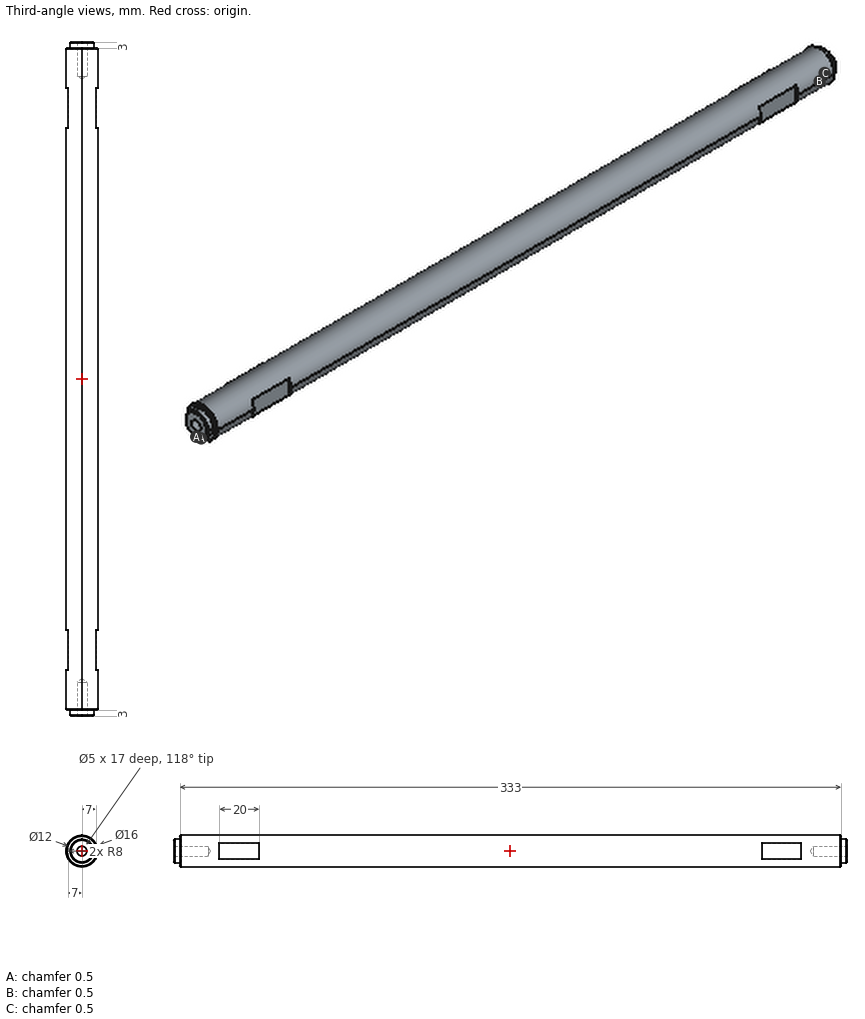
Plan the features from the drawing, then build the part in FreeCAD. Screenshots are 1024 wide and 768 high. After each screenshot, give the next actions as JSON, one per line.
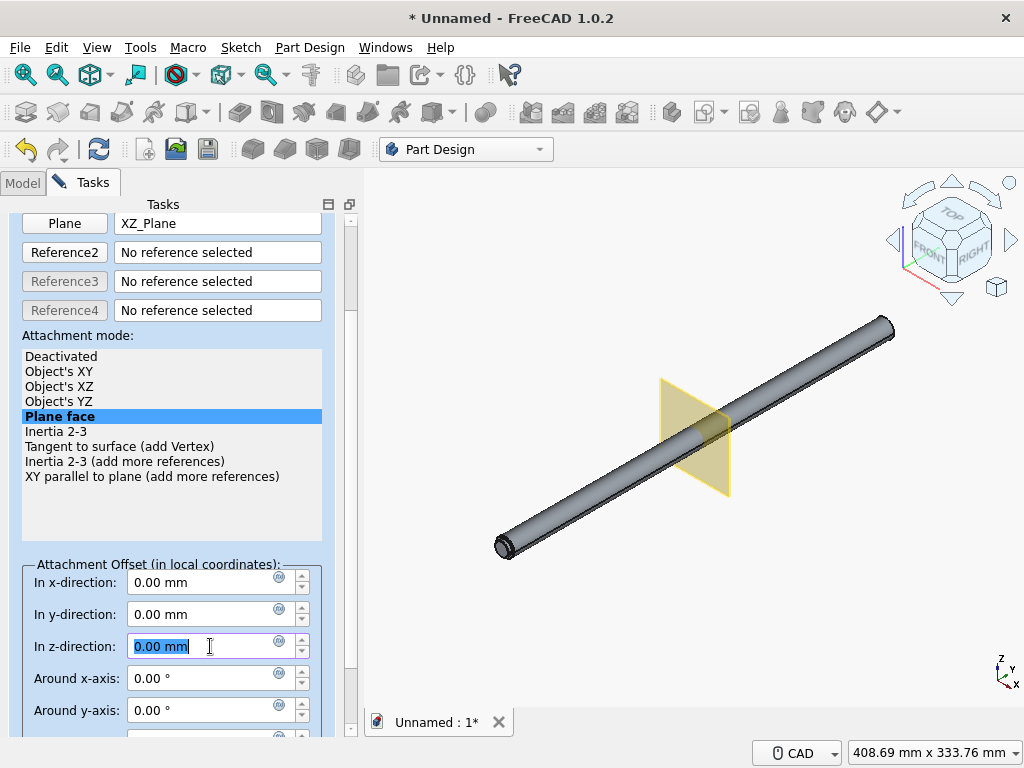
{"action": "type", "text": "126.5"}
{"action": "key", "text": "Tab"}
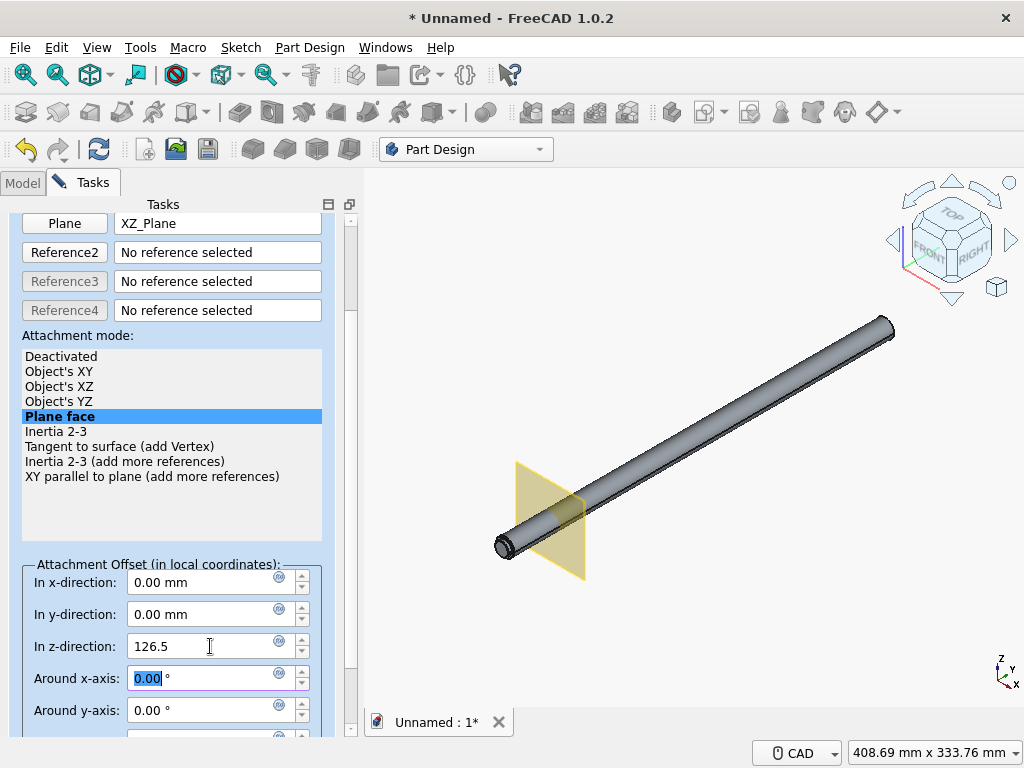
{"action": "scroll", "coordinate": [351, 475], "scroll_direction": "up", "scroll_amount": 3}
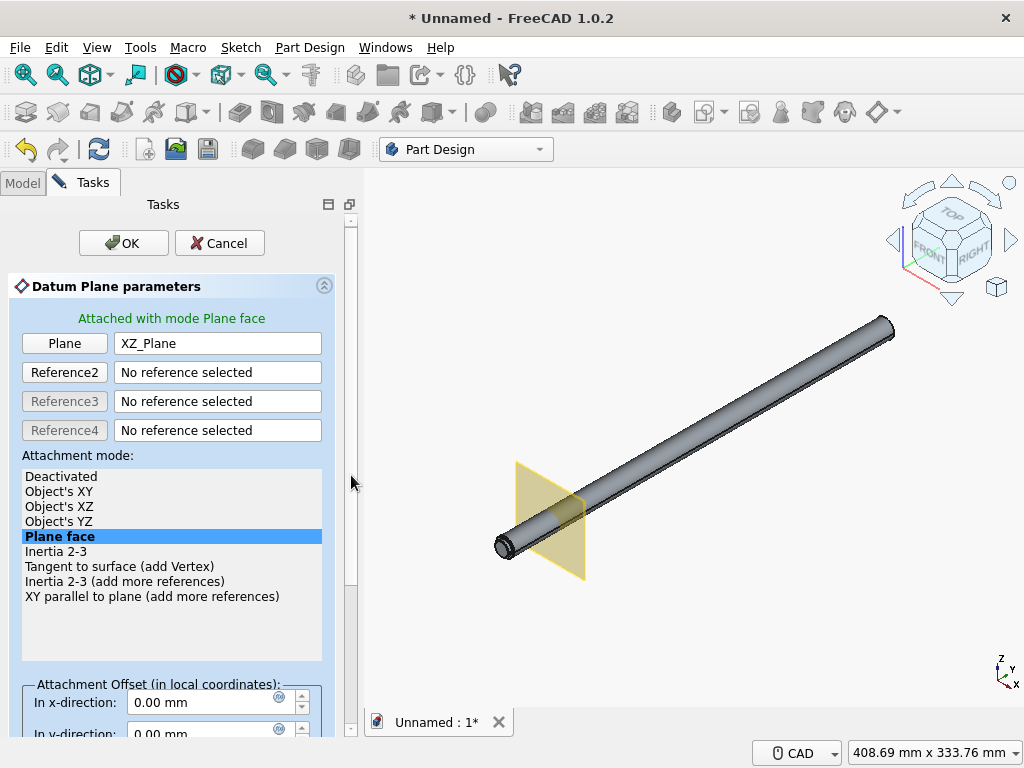
{"action": "left_click", "coordinate": [124, 243]}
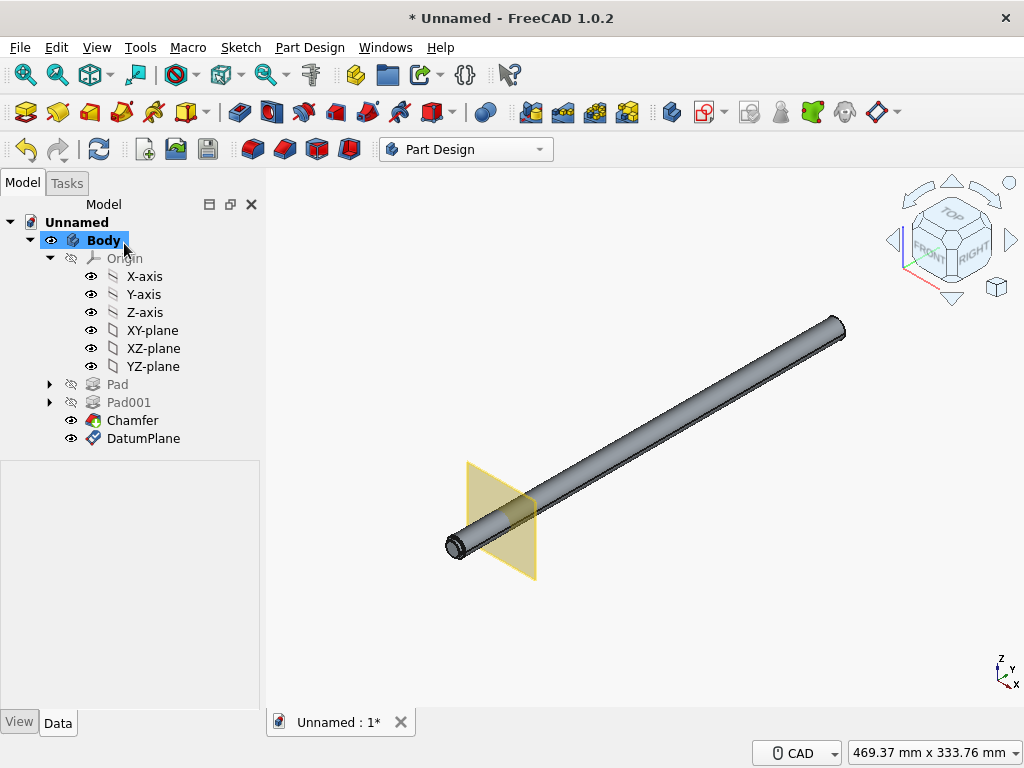
{"action": "left_click", "coordinate": [116, 438]}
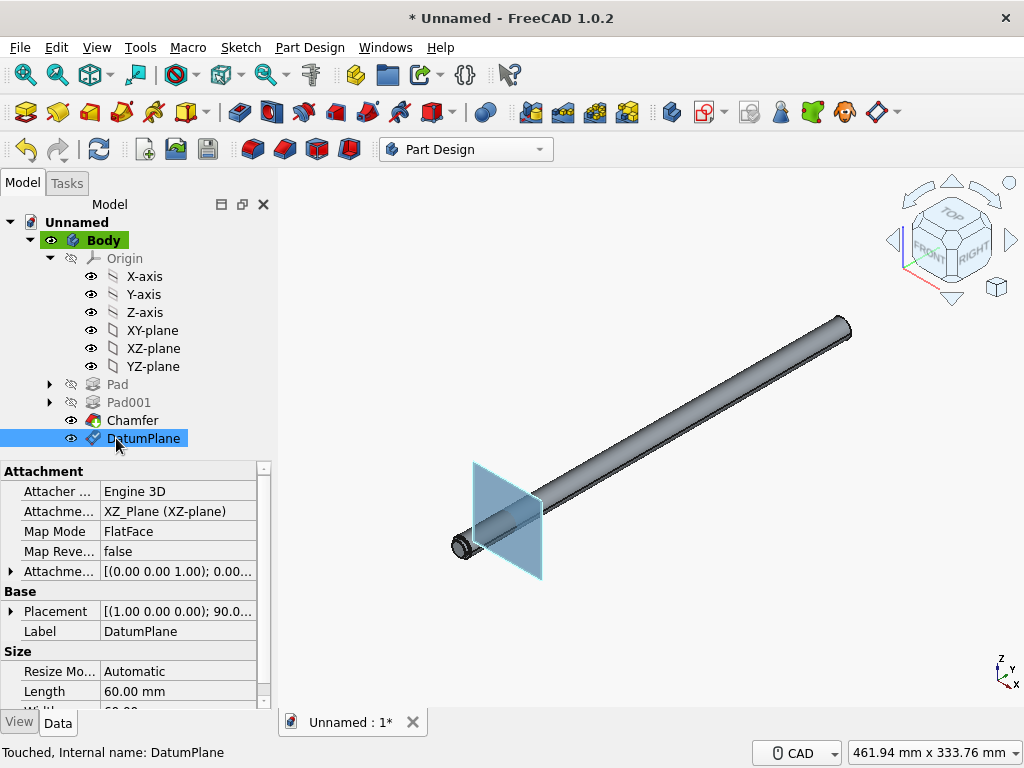
{"action": "left_click", "coordinate": [704, 112]}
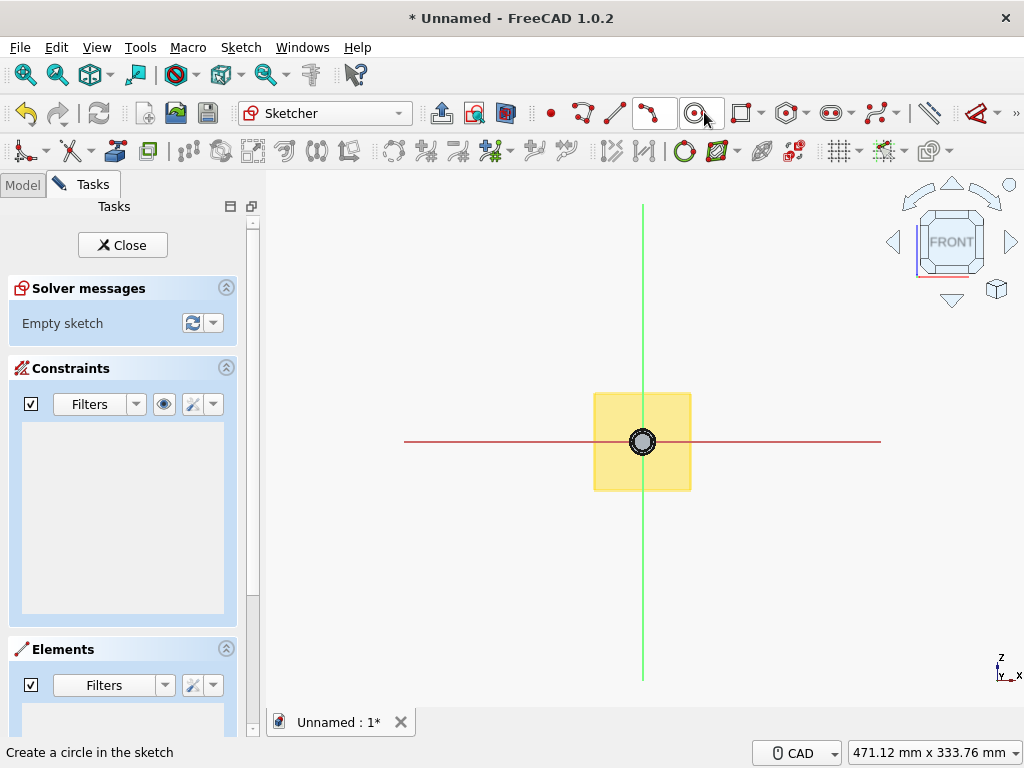
{"action": "key", "text": "q s"}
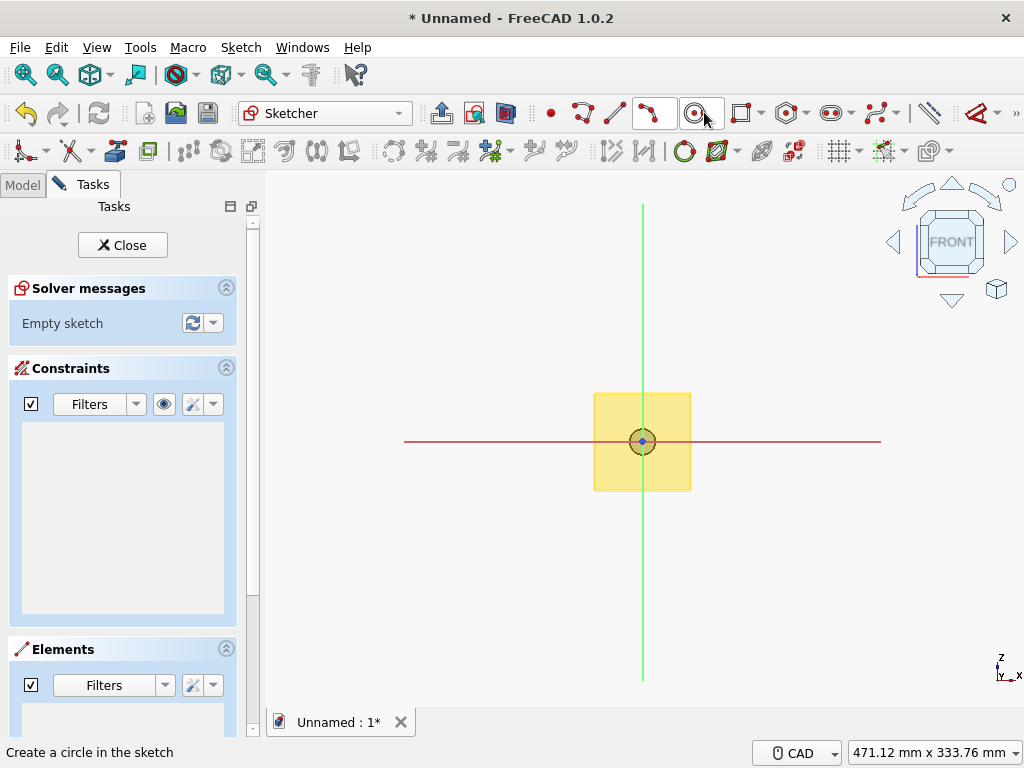
{"action": "scroll", "coordinate": [647, 442], "scroll_direction": "up", "scroll_amount": 14}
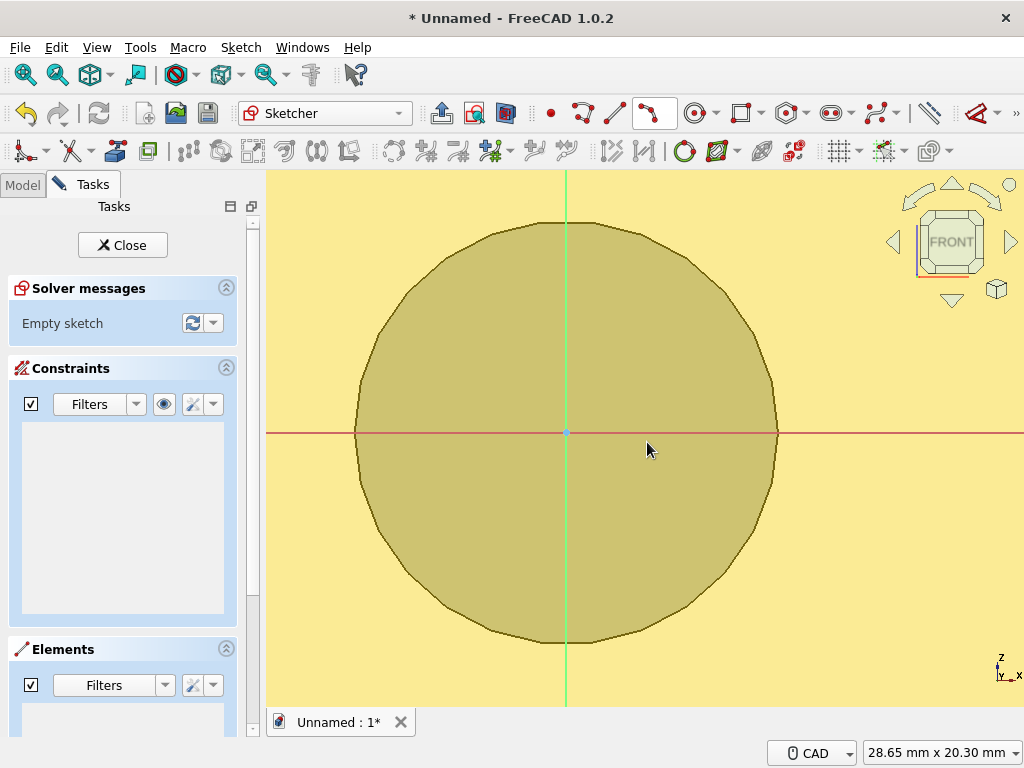
{"action": "left_click", "coordinate": [616, 114]}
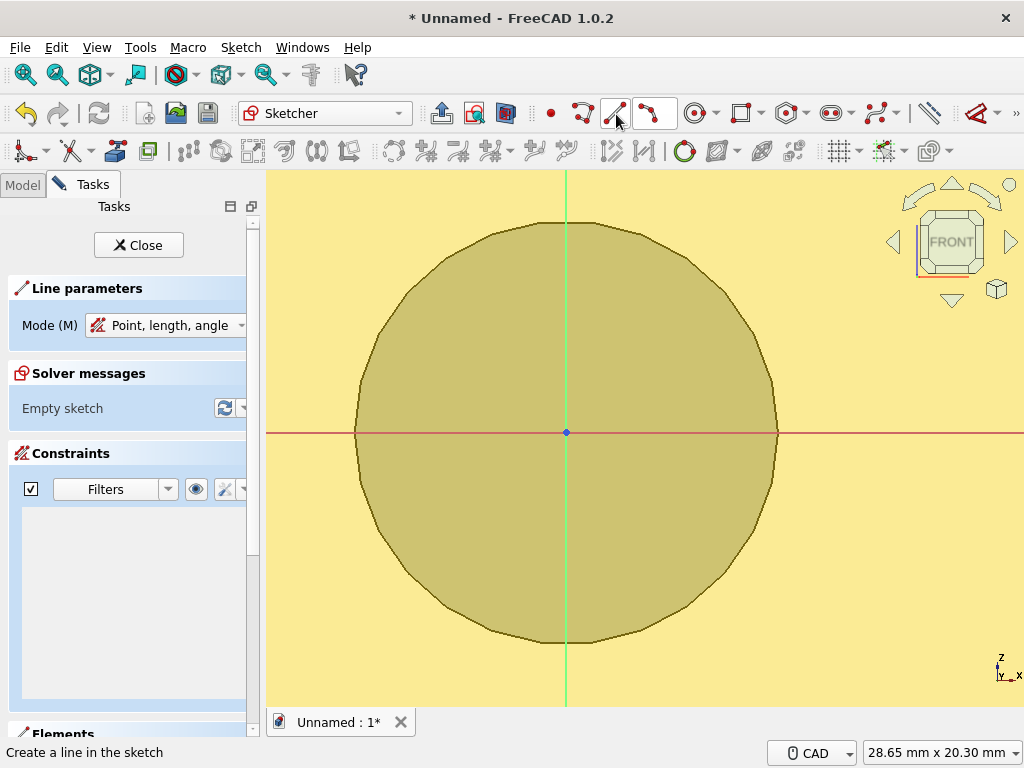
{"action": "left_click", "coordinate": [381, 535]}
{"action": "left_click", "coordinate": [381, 330]}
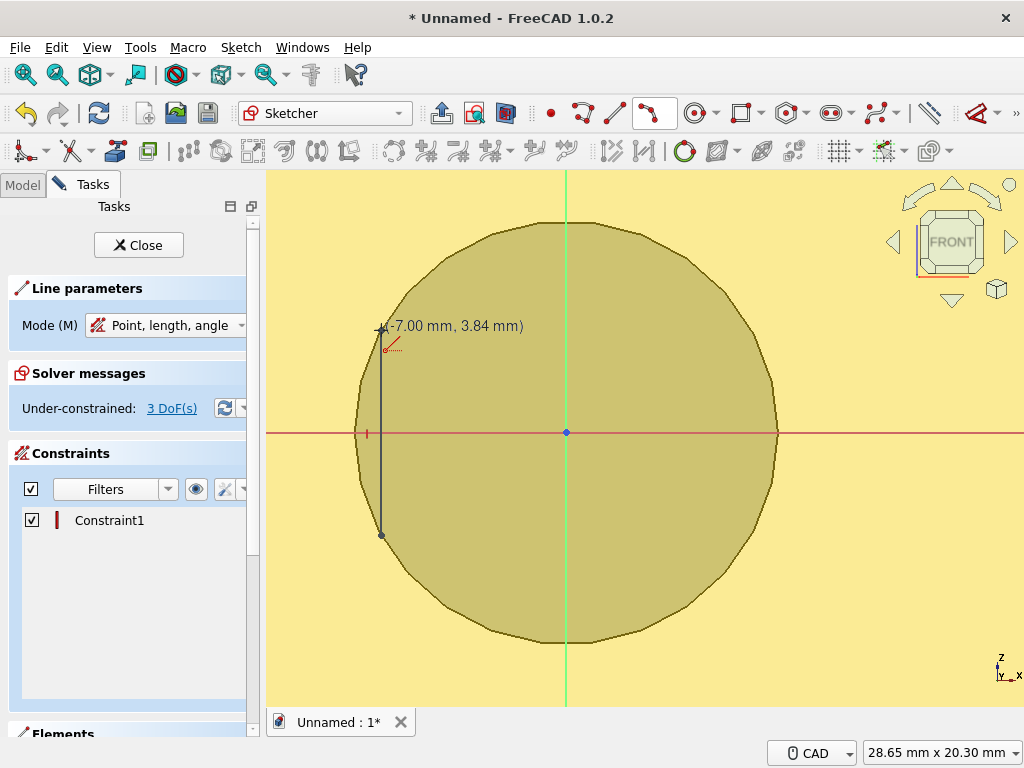
{"action": "key", "text": "g 3 a"}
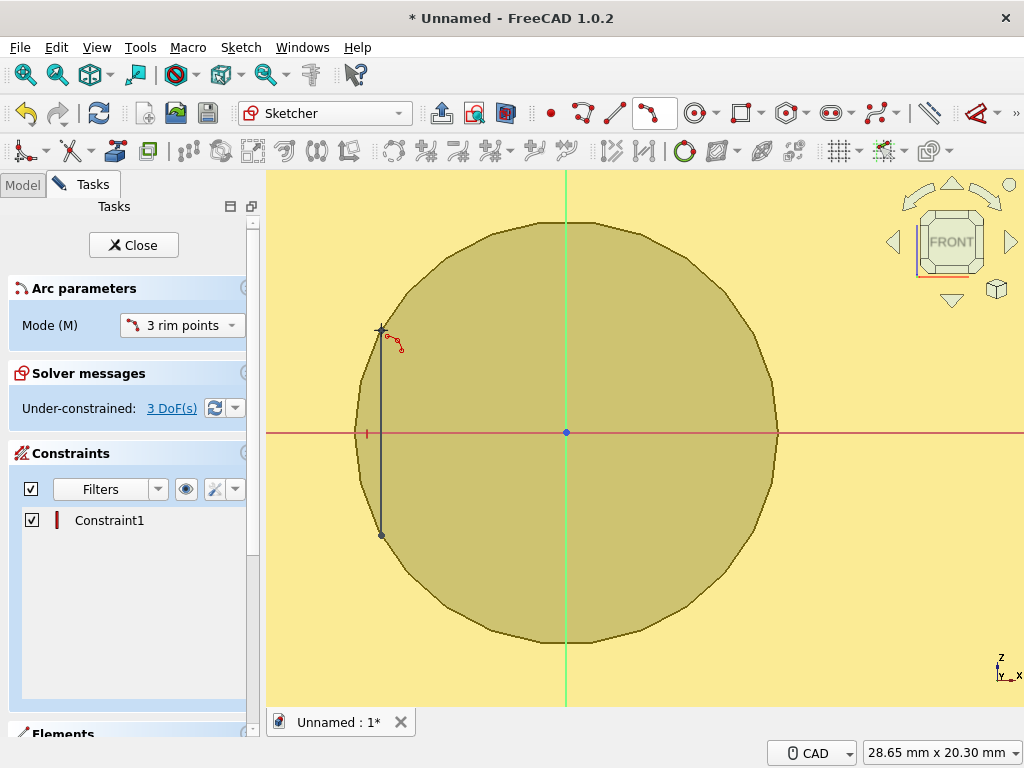
{"action": "left_click", "coordinate": [381, 331]}
{"action": "left_click", "coordinate": [381, 536]}
{"action": "left_click", "coordinate": [356, 411]}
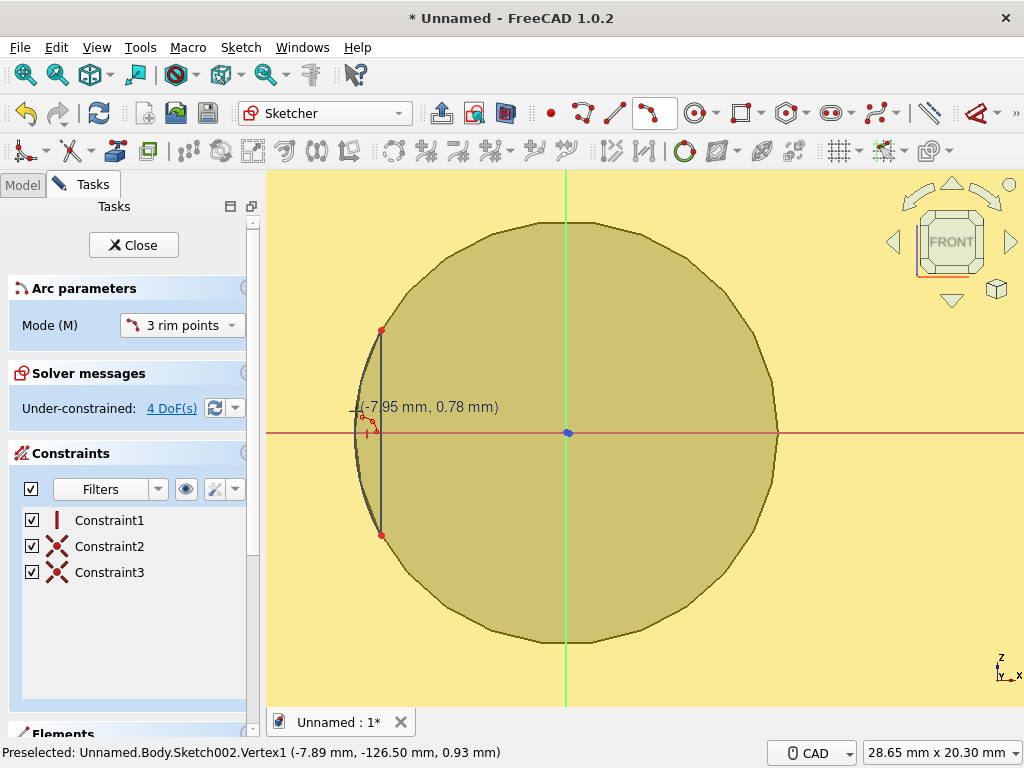
{"action": "key", "text": "g l"}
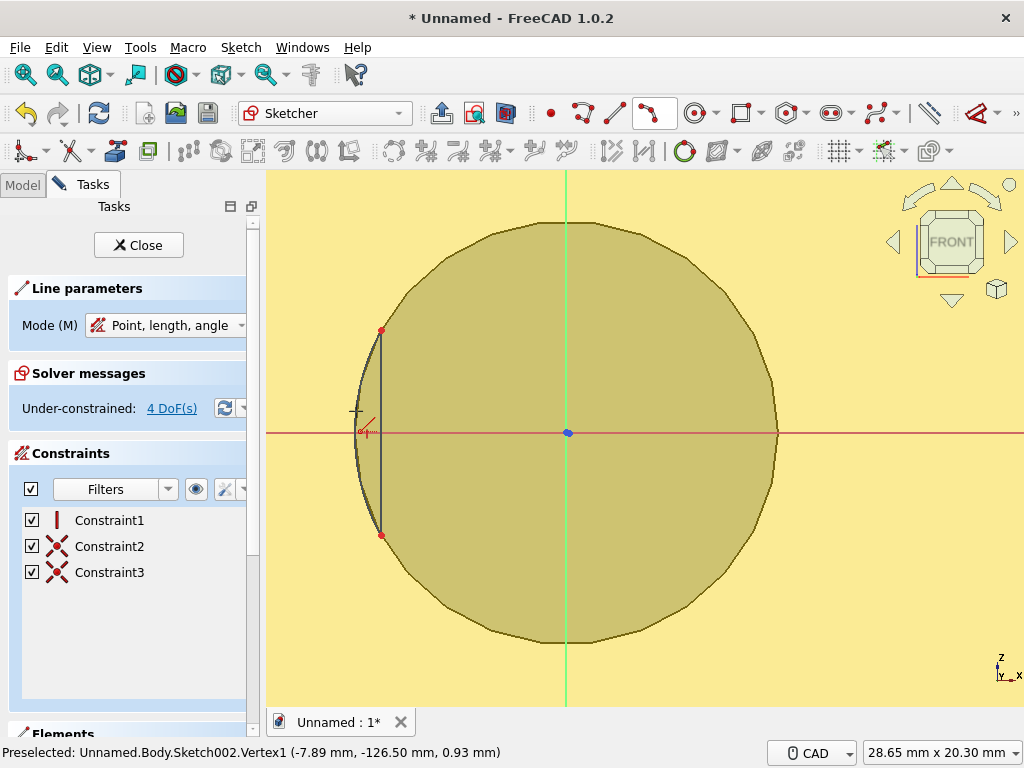
{"action": "left_click", "coordinate": [752, 330]}
{"action": "left_click", "coordinate": [752, 535]}